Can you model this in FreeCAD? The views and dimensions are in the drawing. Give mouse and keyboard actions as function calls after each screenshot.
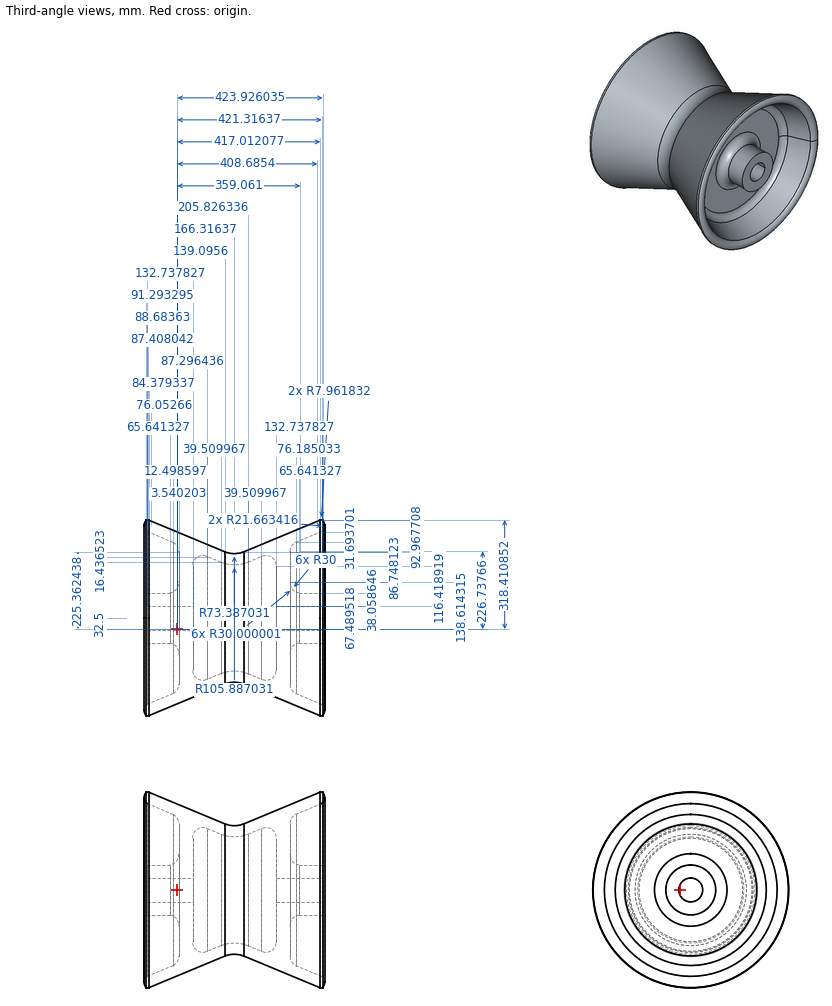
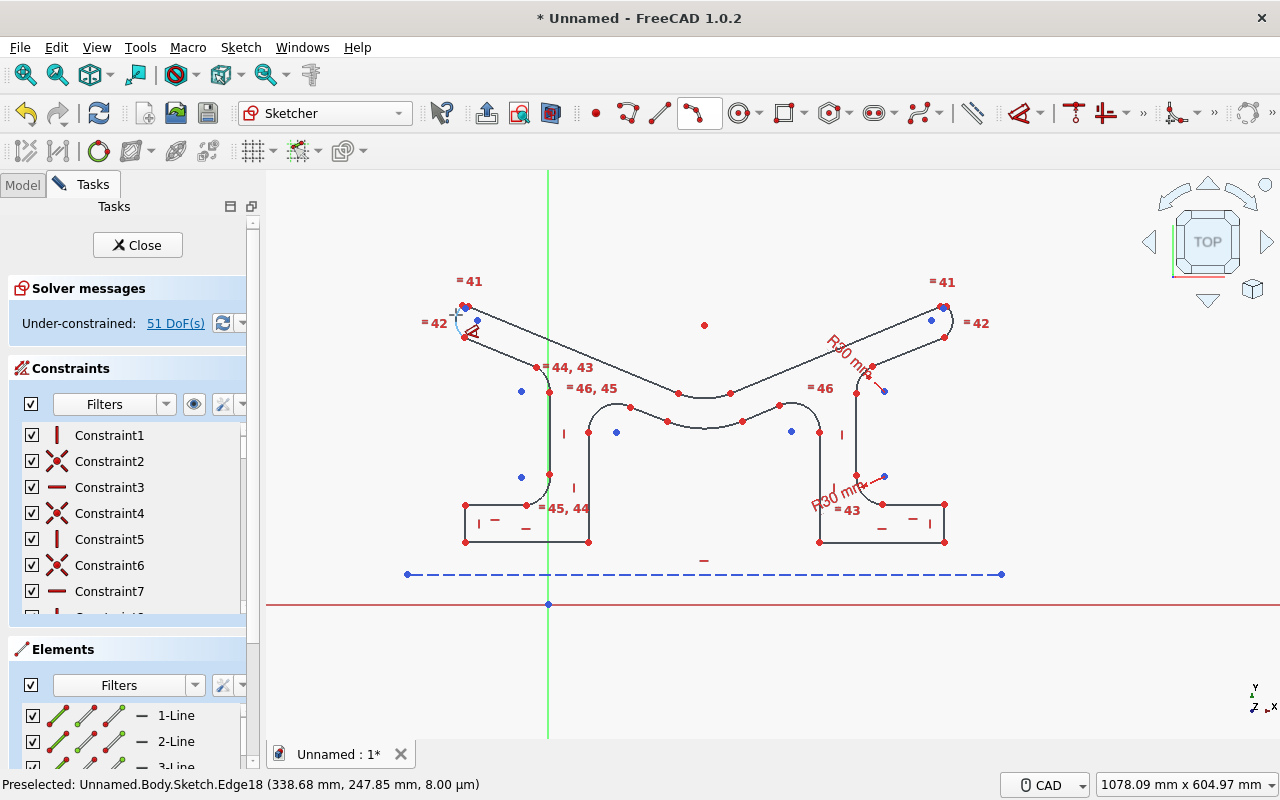
scroll(951, 329, up, 4)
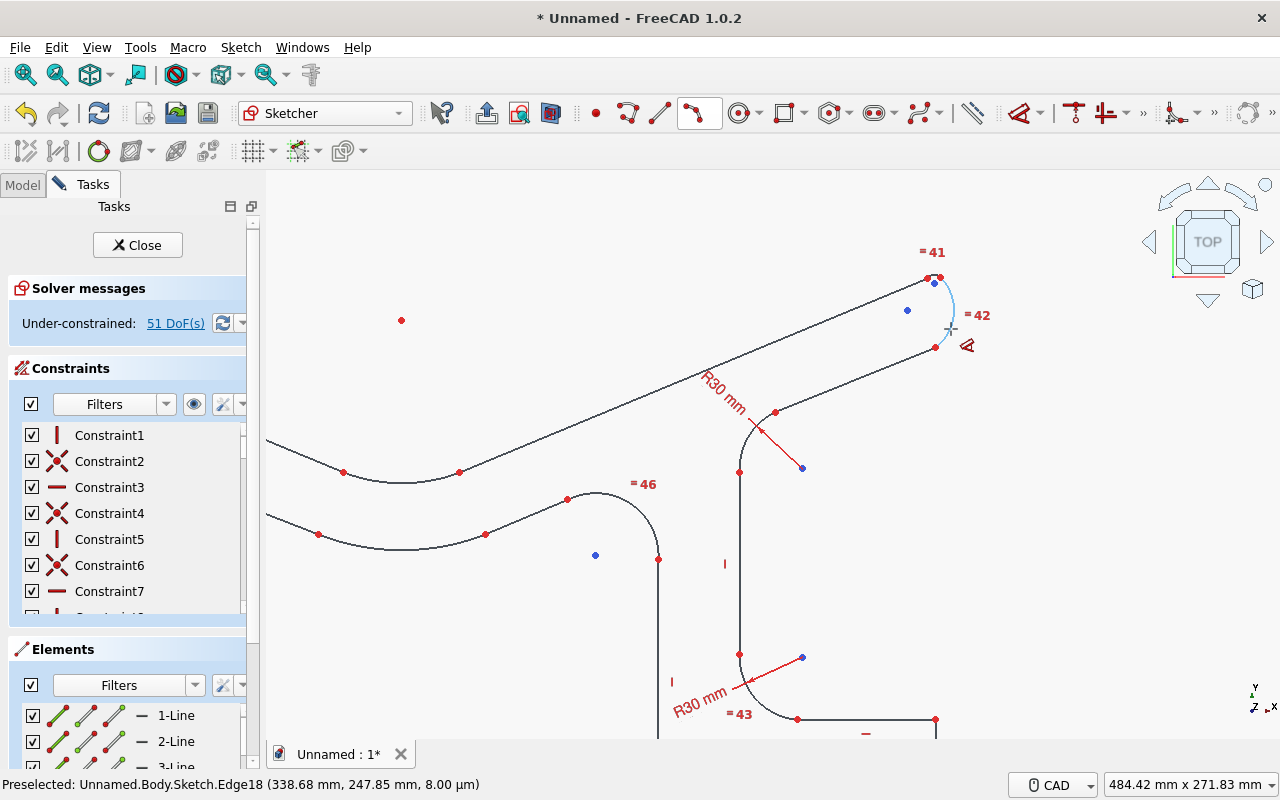
click(950, 329)
click(979, 342)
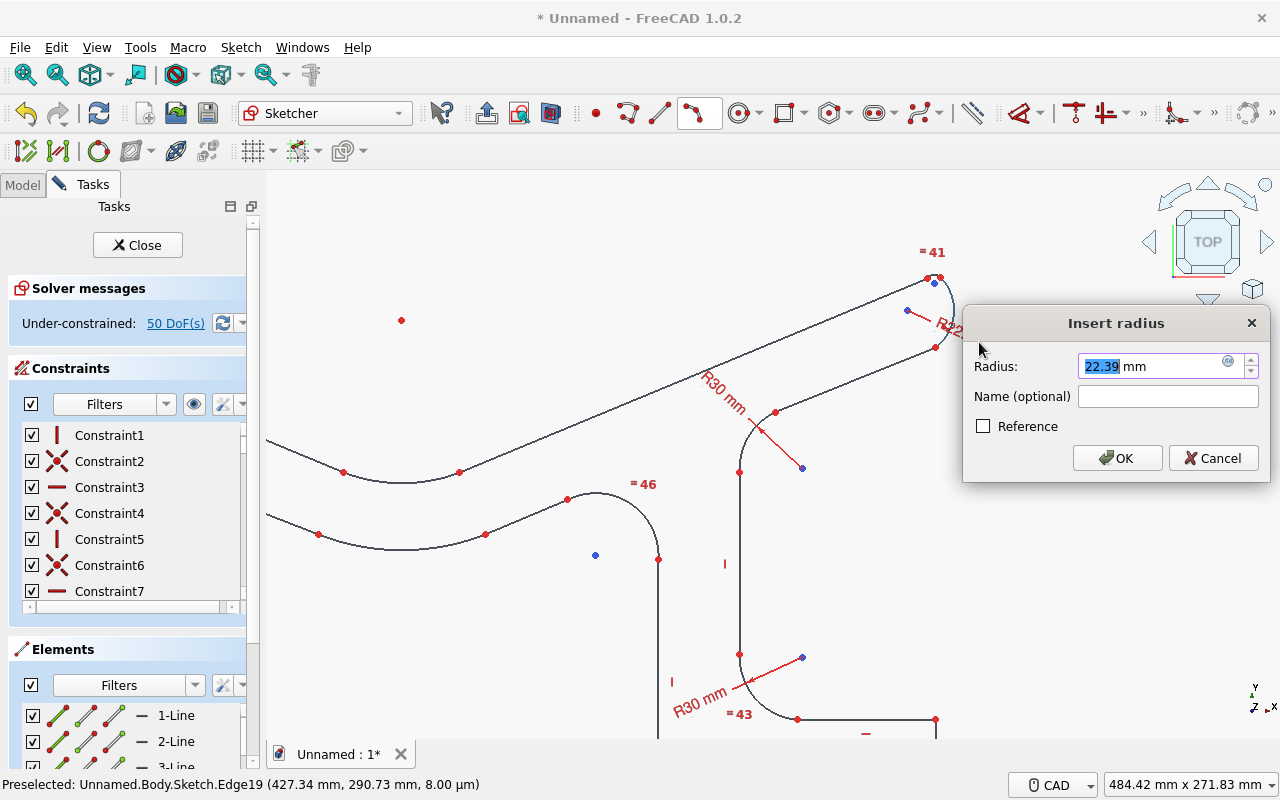
text(21.663416)
key(Return)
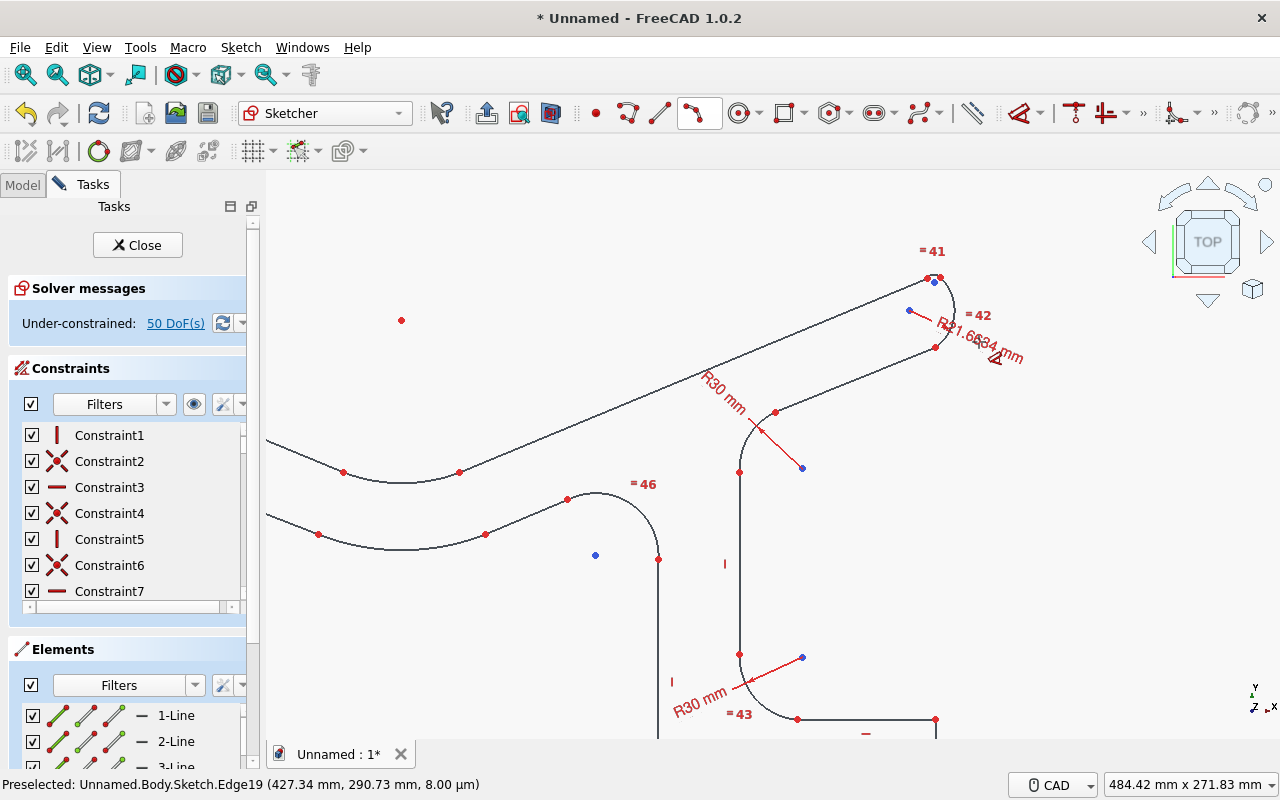
scroll(933, 275, up, 5)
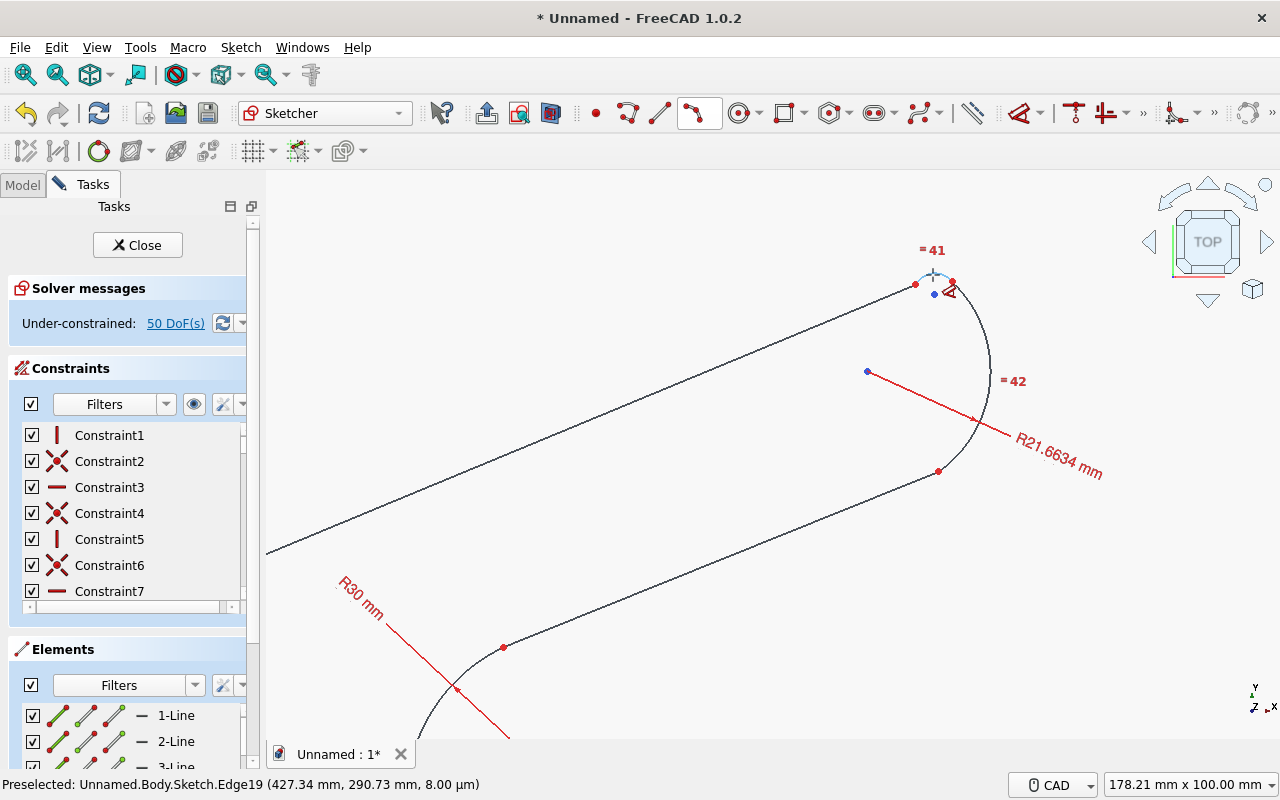
click(933, 273)
click(930, 241)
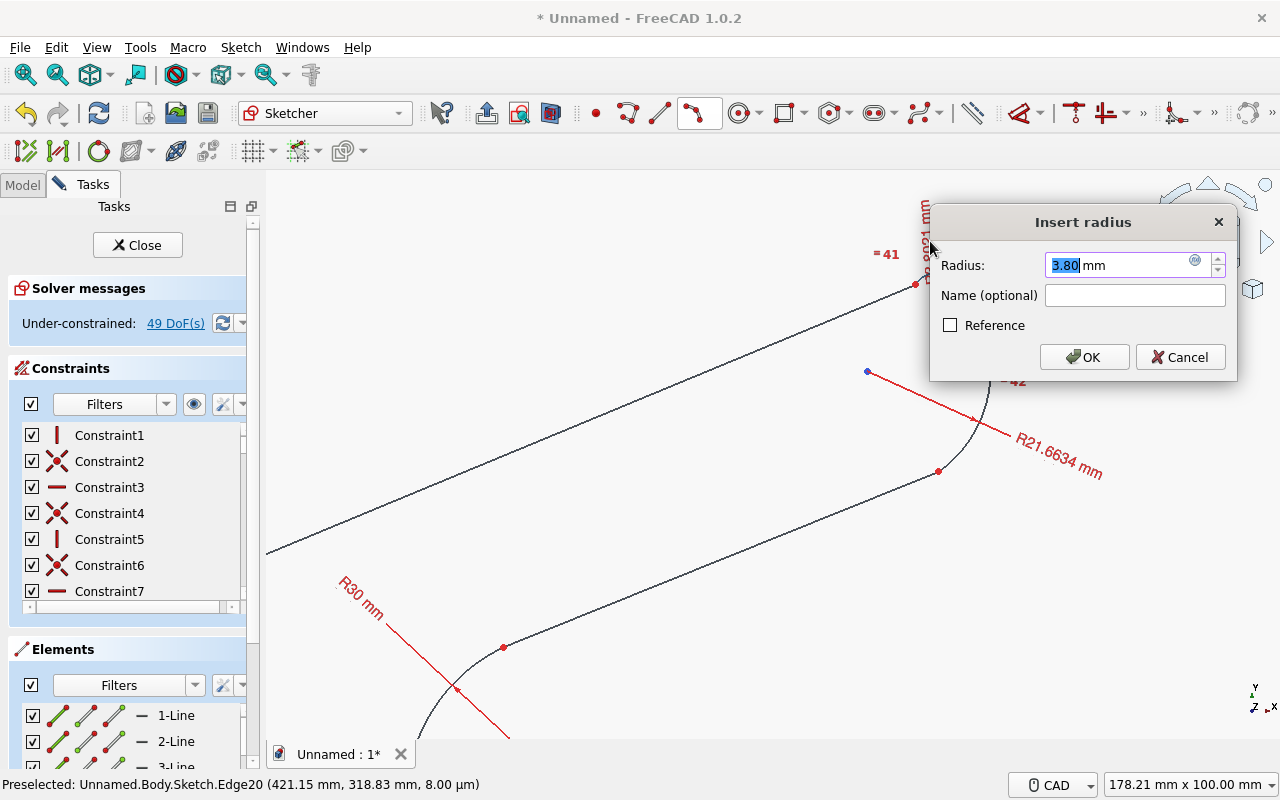
text(7.961832)
key(Return)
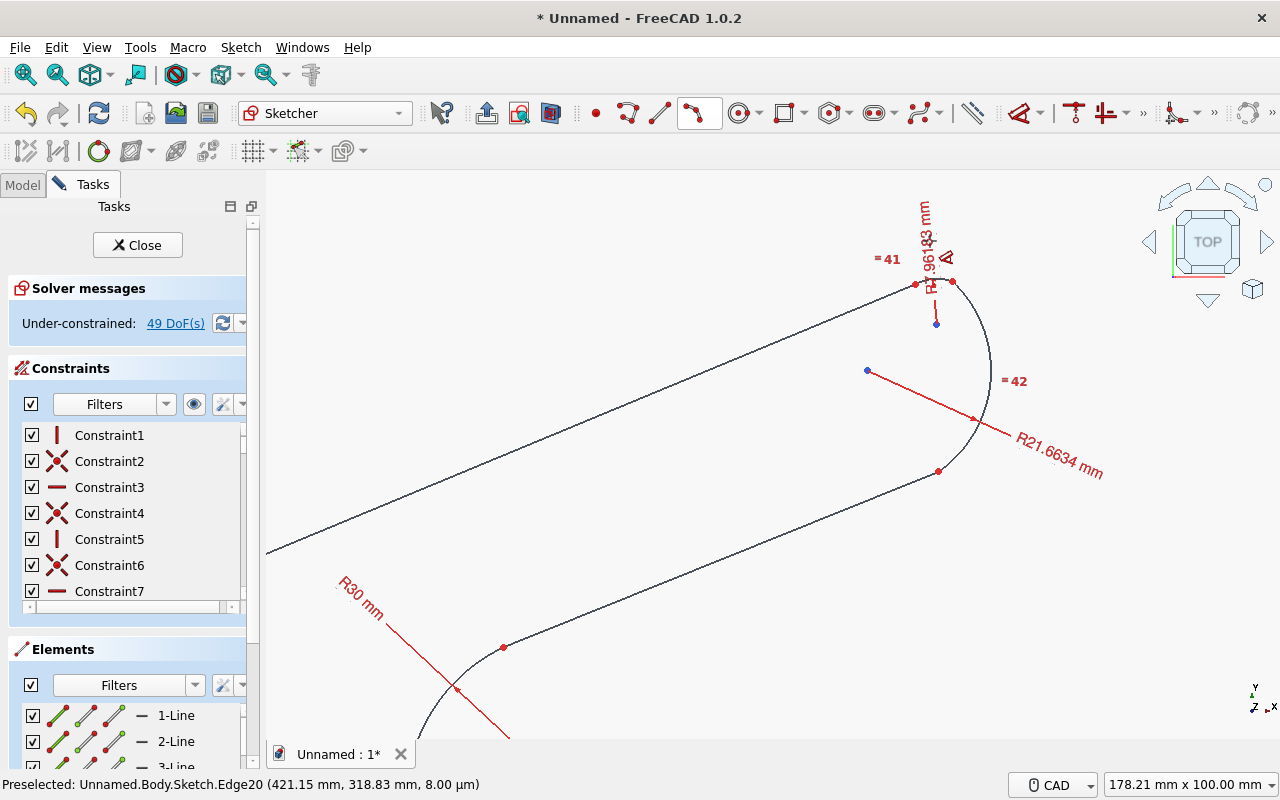
scroll(946, 311, down, 9)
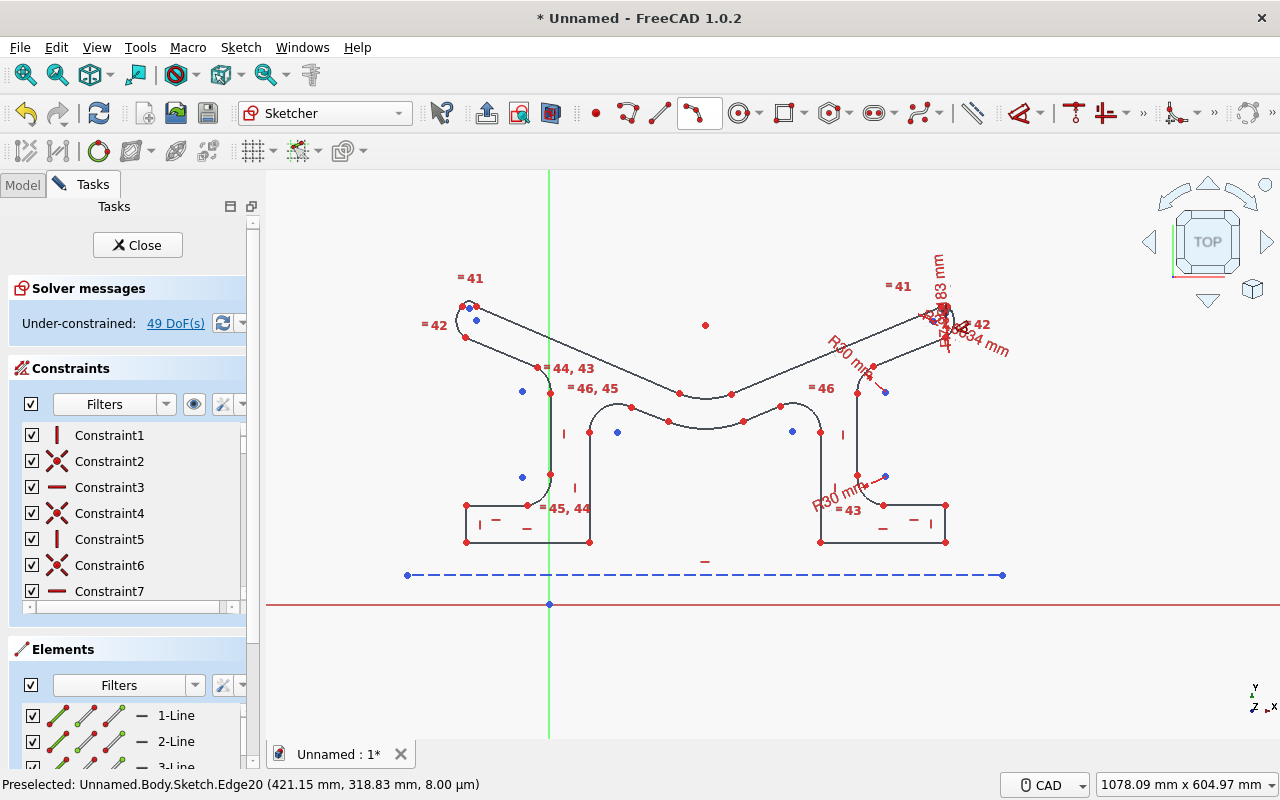
click(695, 398)
click(602, 310)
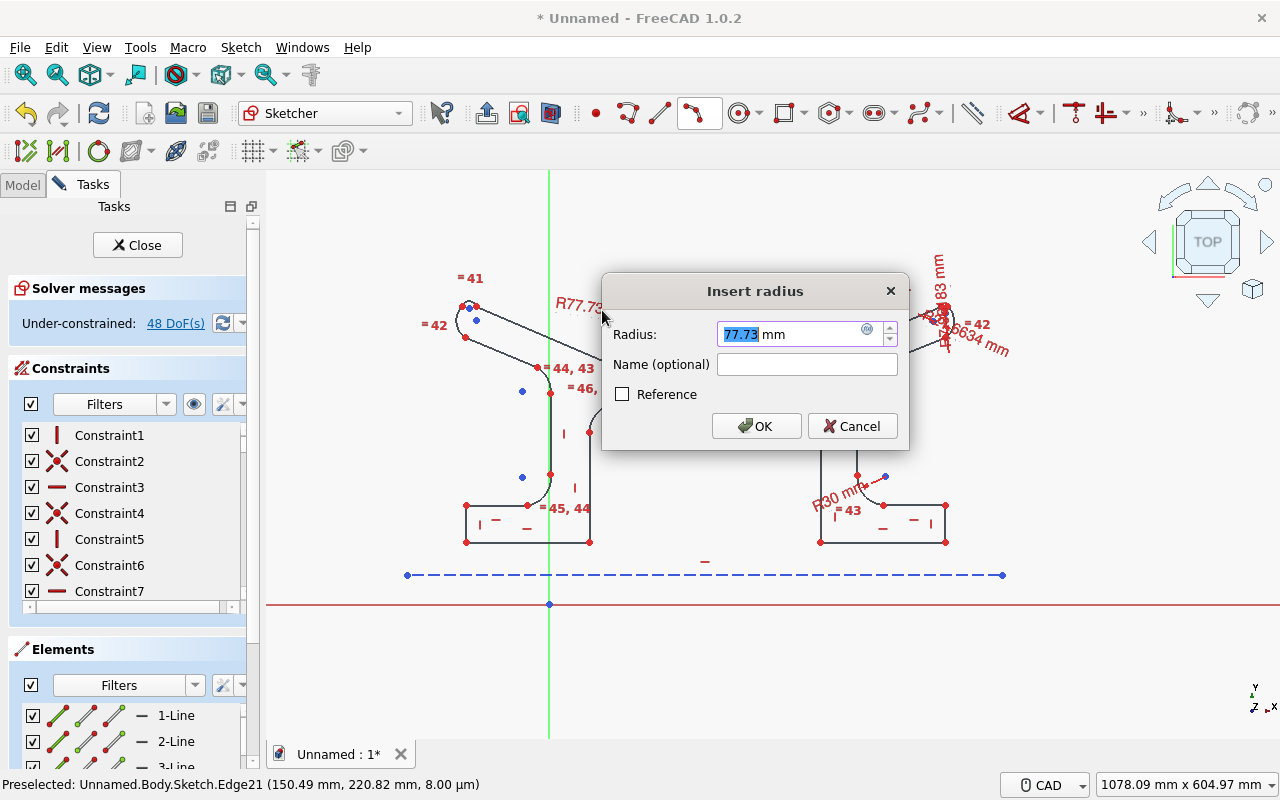
text(73.387031)
key(Return)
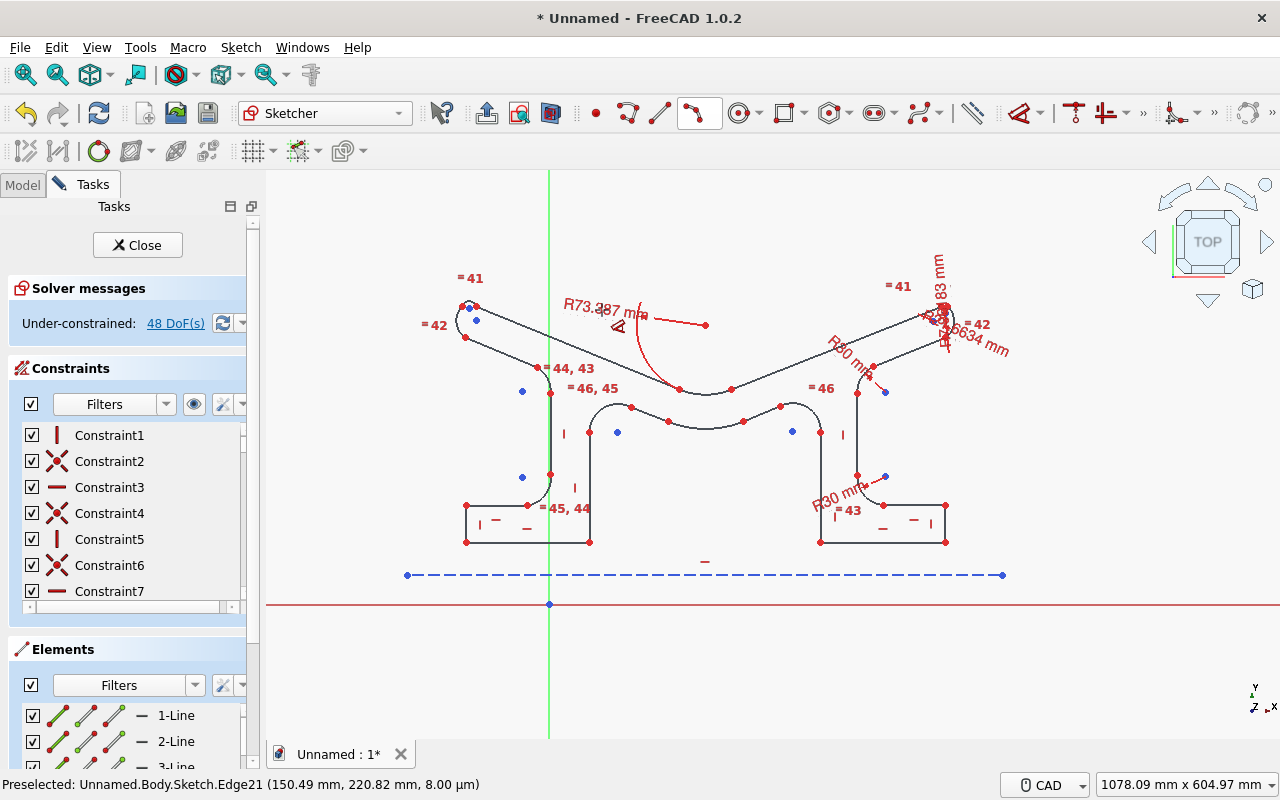
click(690, 428)
click(685, 460)